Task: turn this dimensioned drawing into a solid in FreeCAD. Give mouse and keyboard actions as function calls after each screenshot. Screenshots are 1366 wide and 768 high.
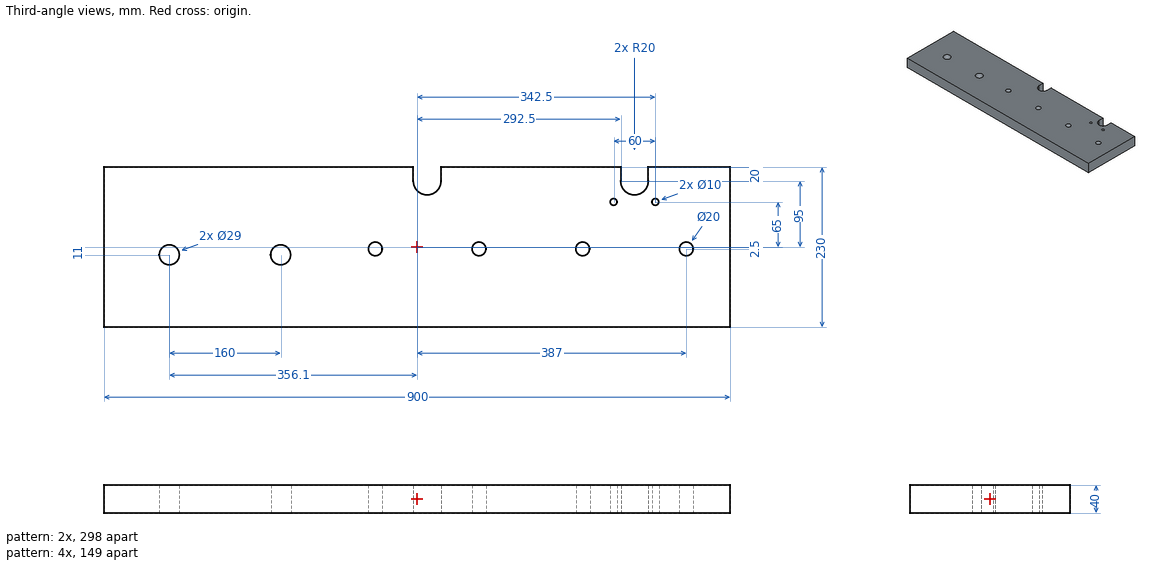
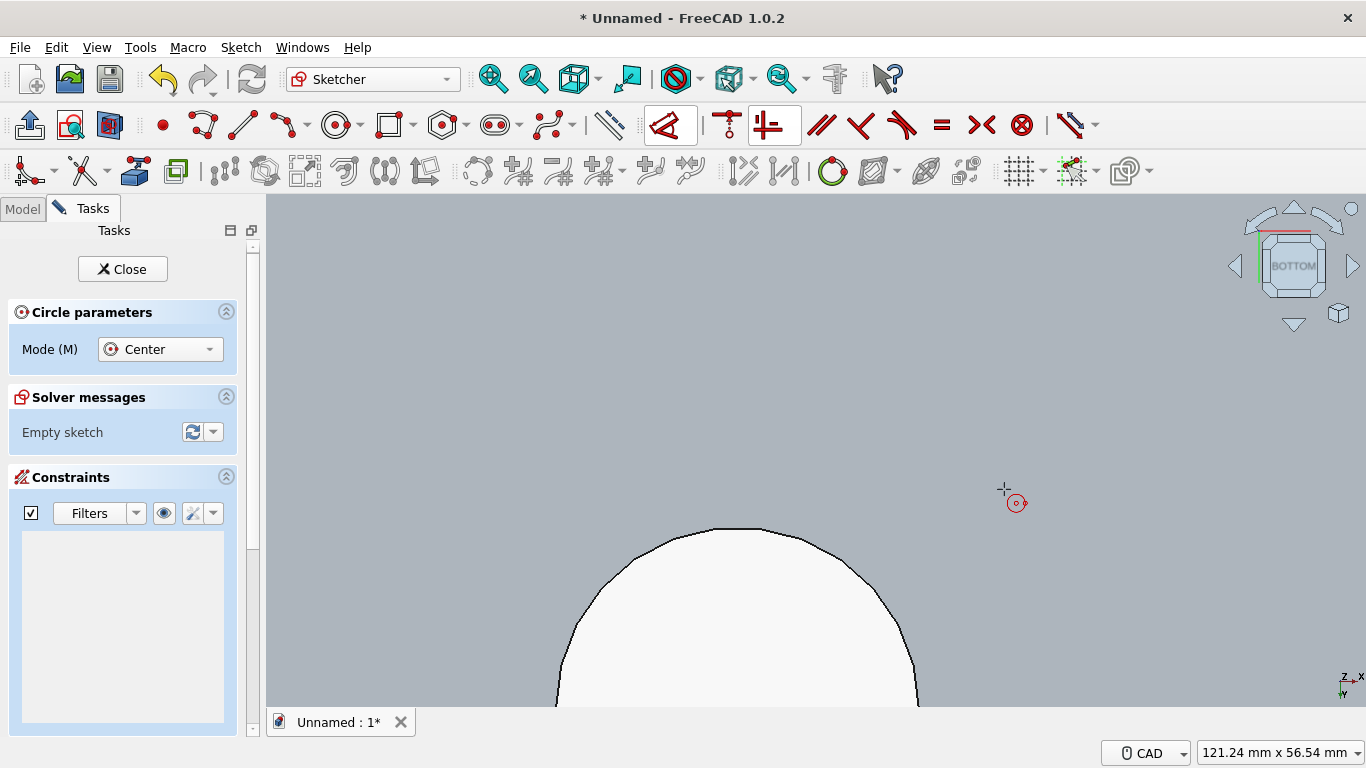
click(1010, 437)
move(1042, 405)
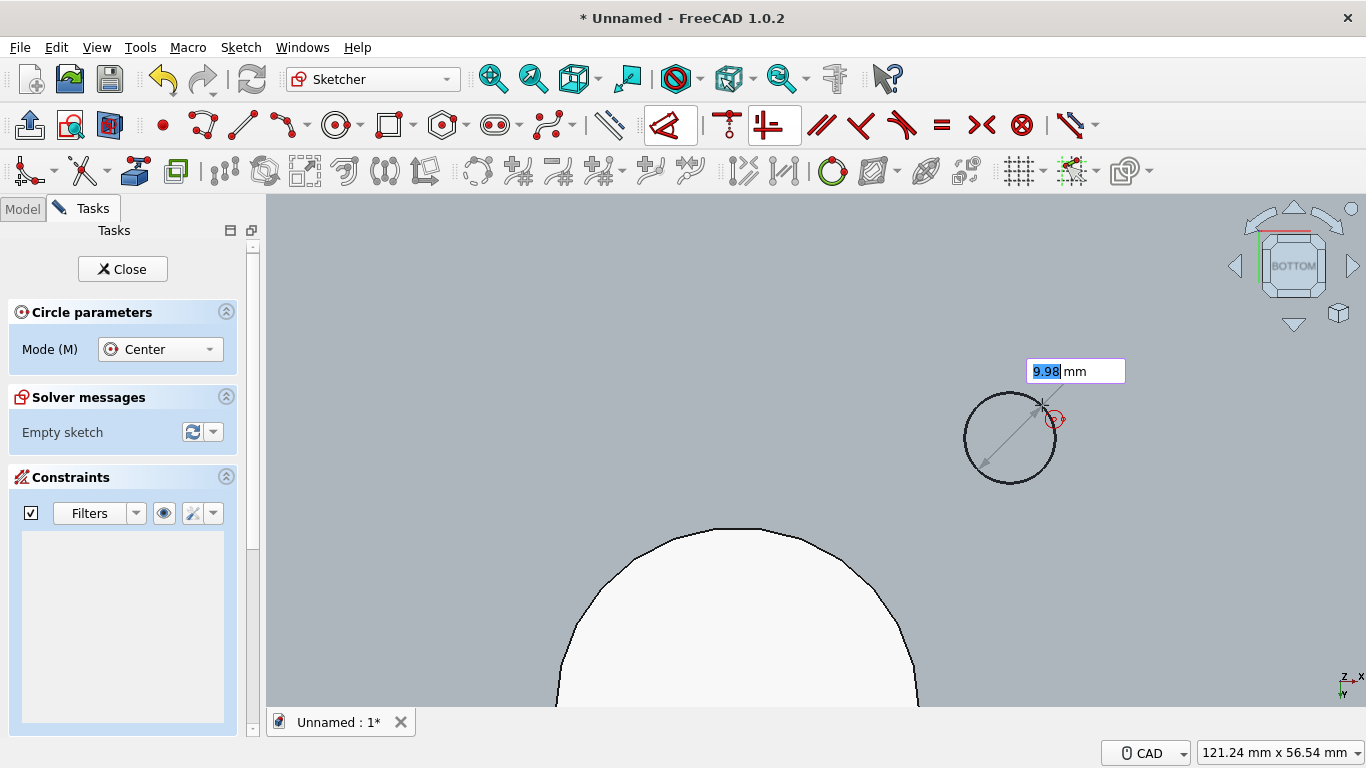
text(10)
key(Return)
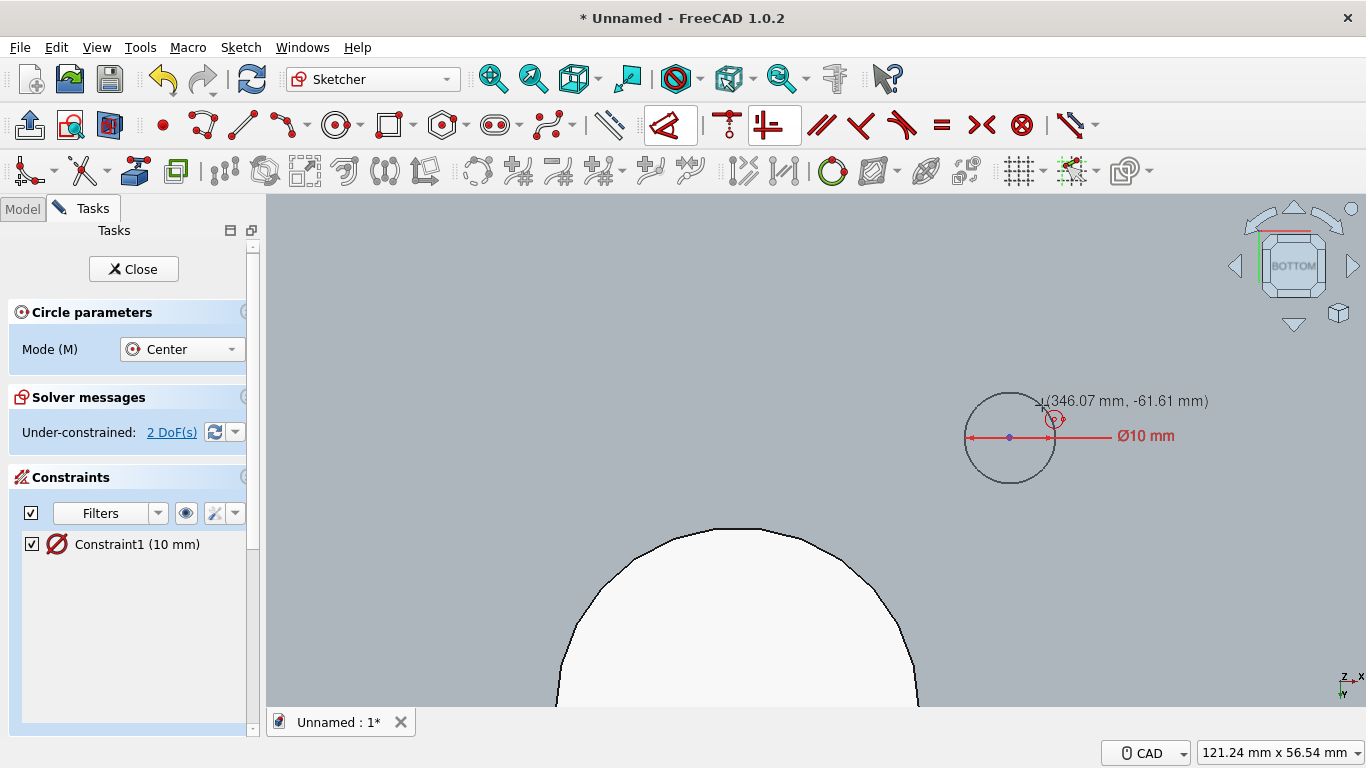
click(465, 437)
move(497, 405)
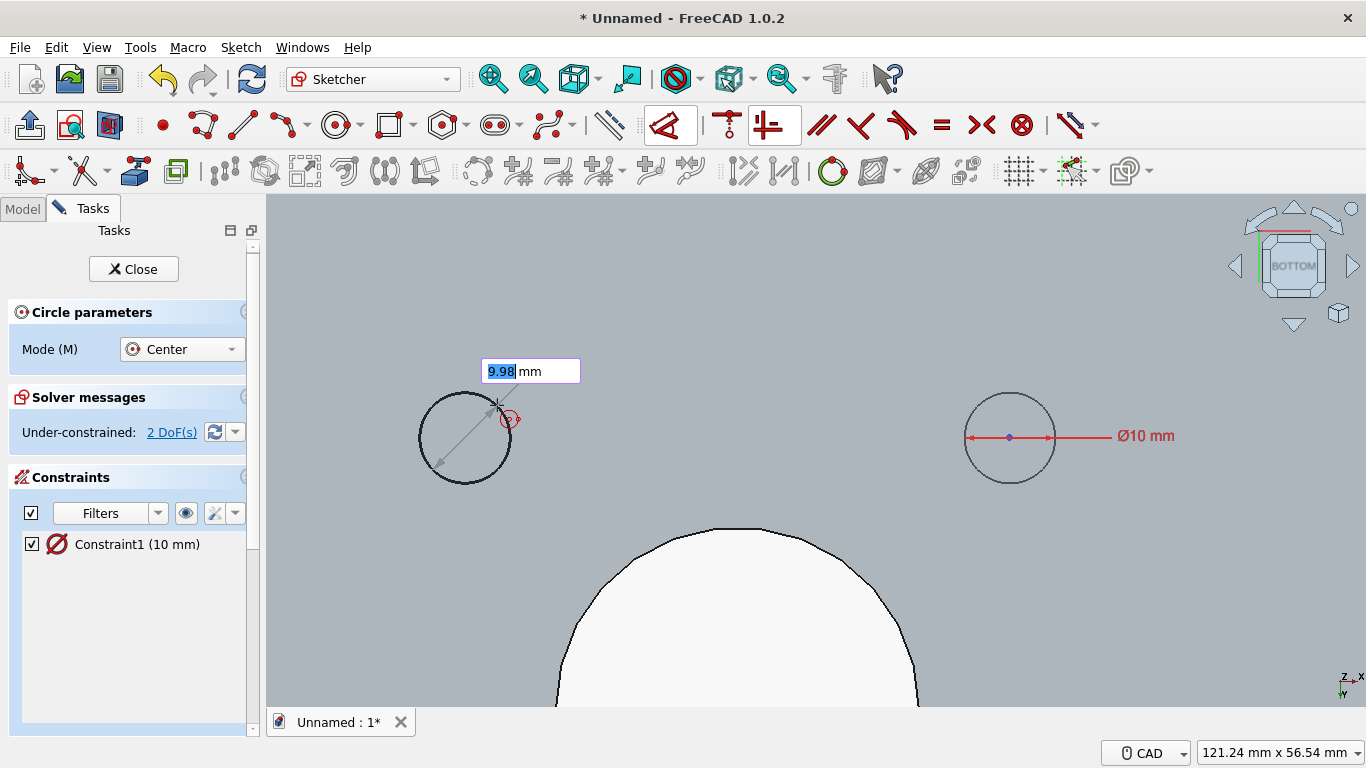
text(10)
key(Return)
key(Escape)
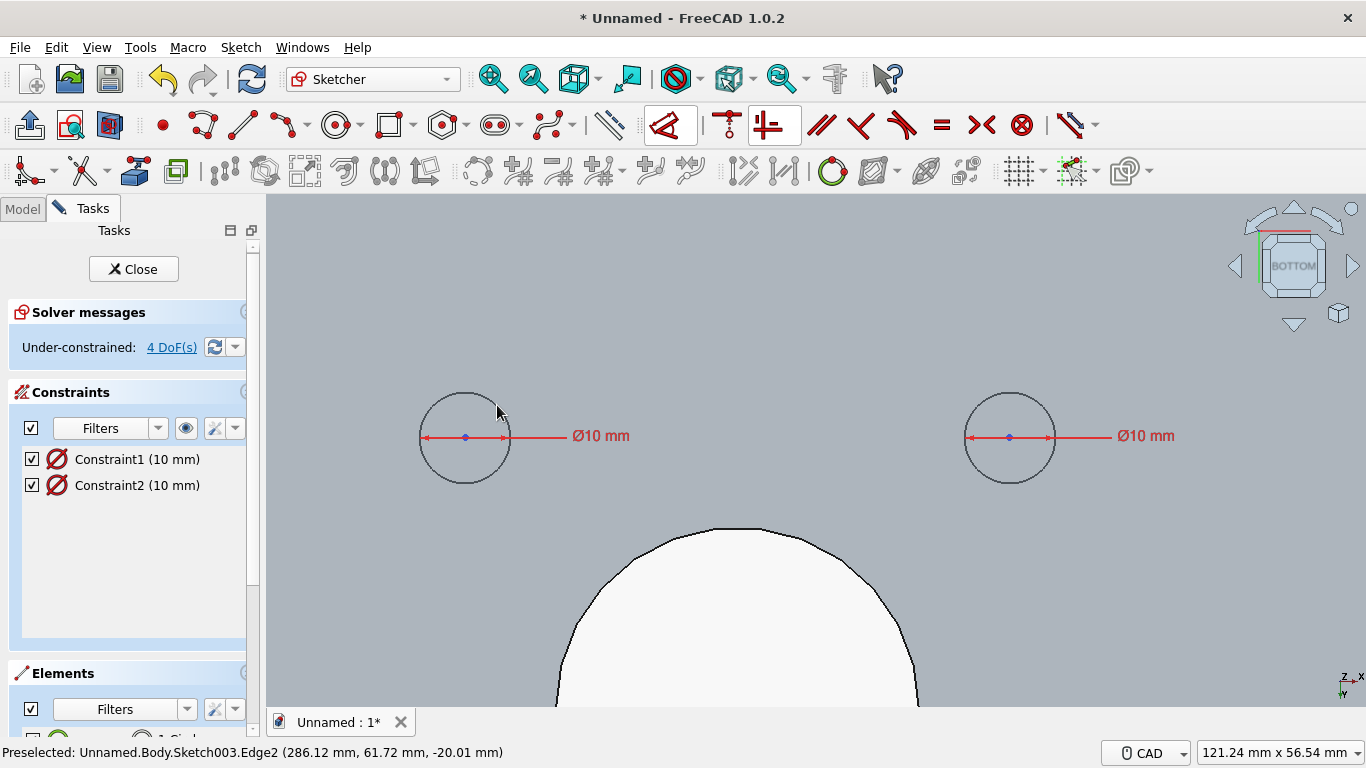
click(1010, 438)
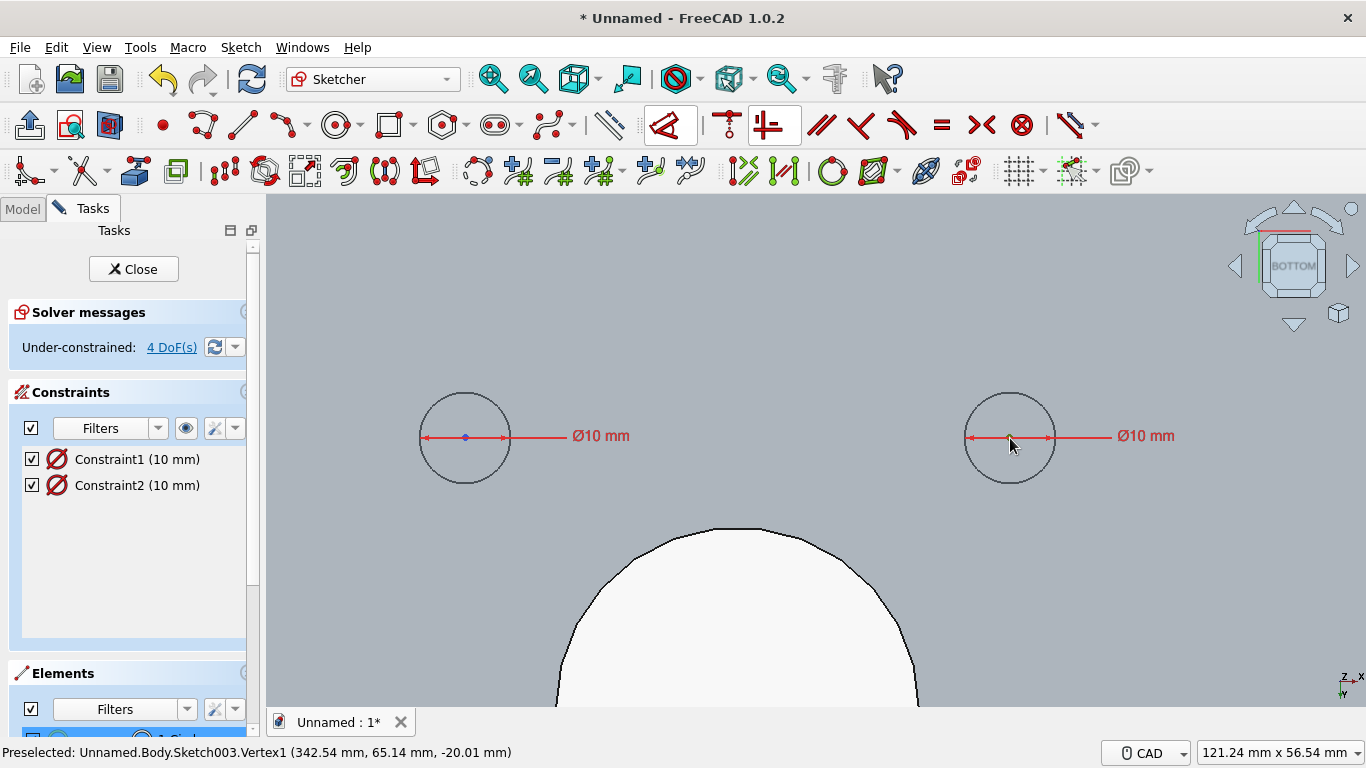
click(465, 438)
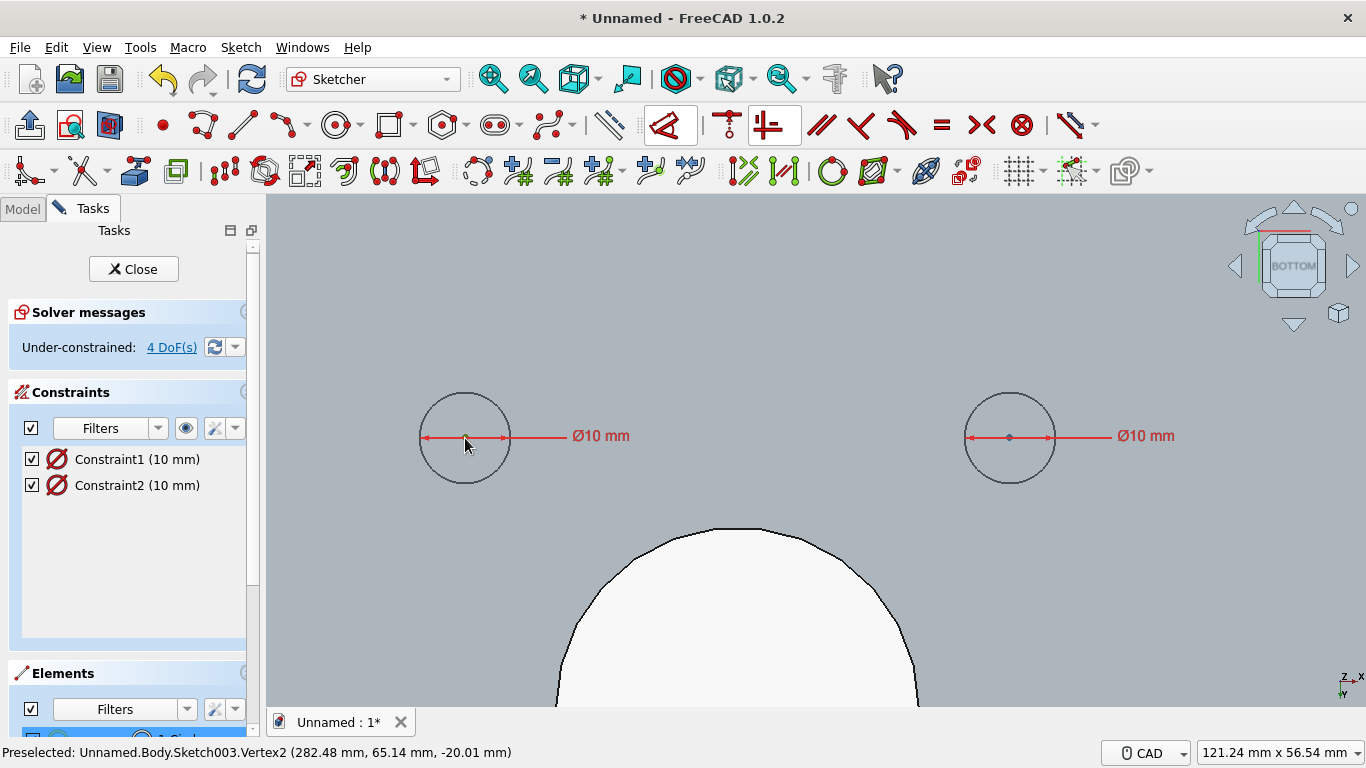
click(796, 126)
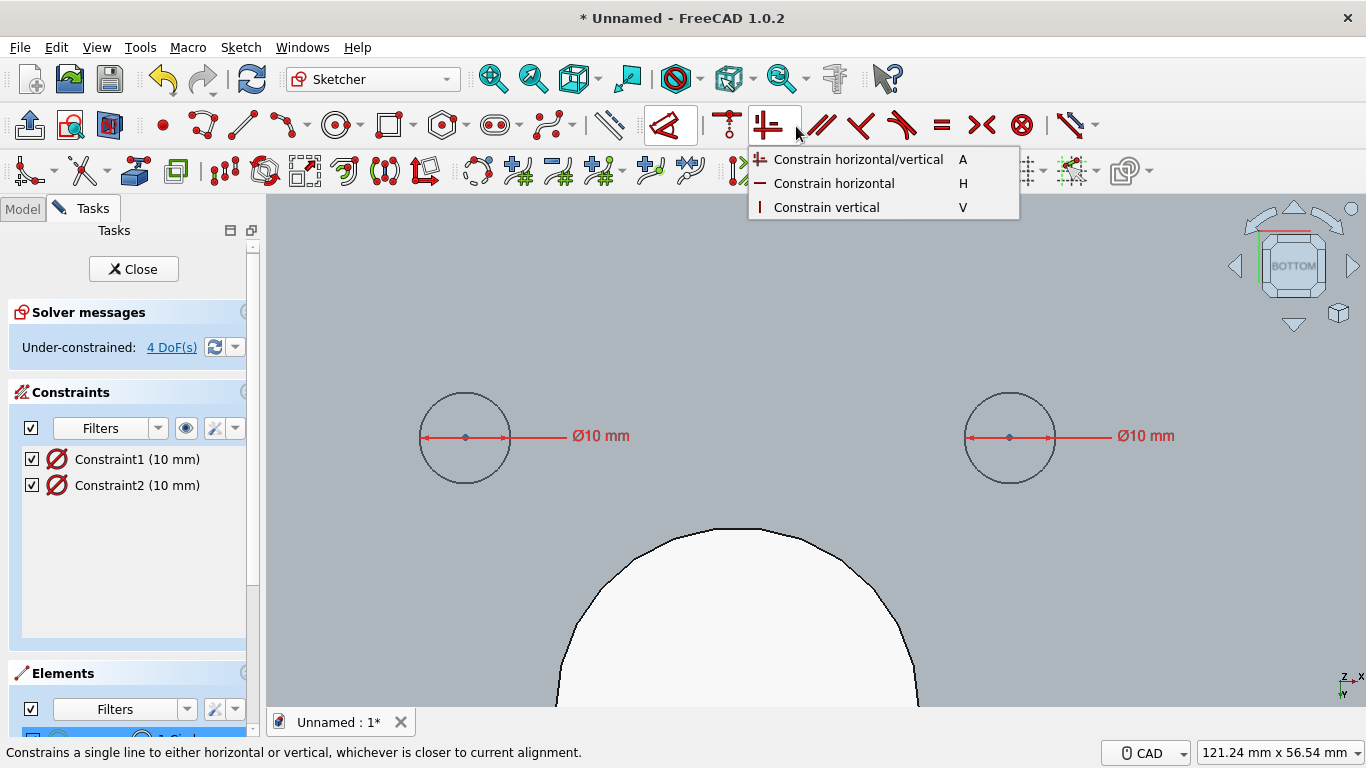
click(884, 183)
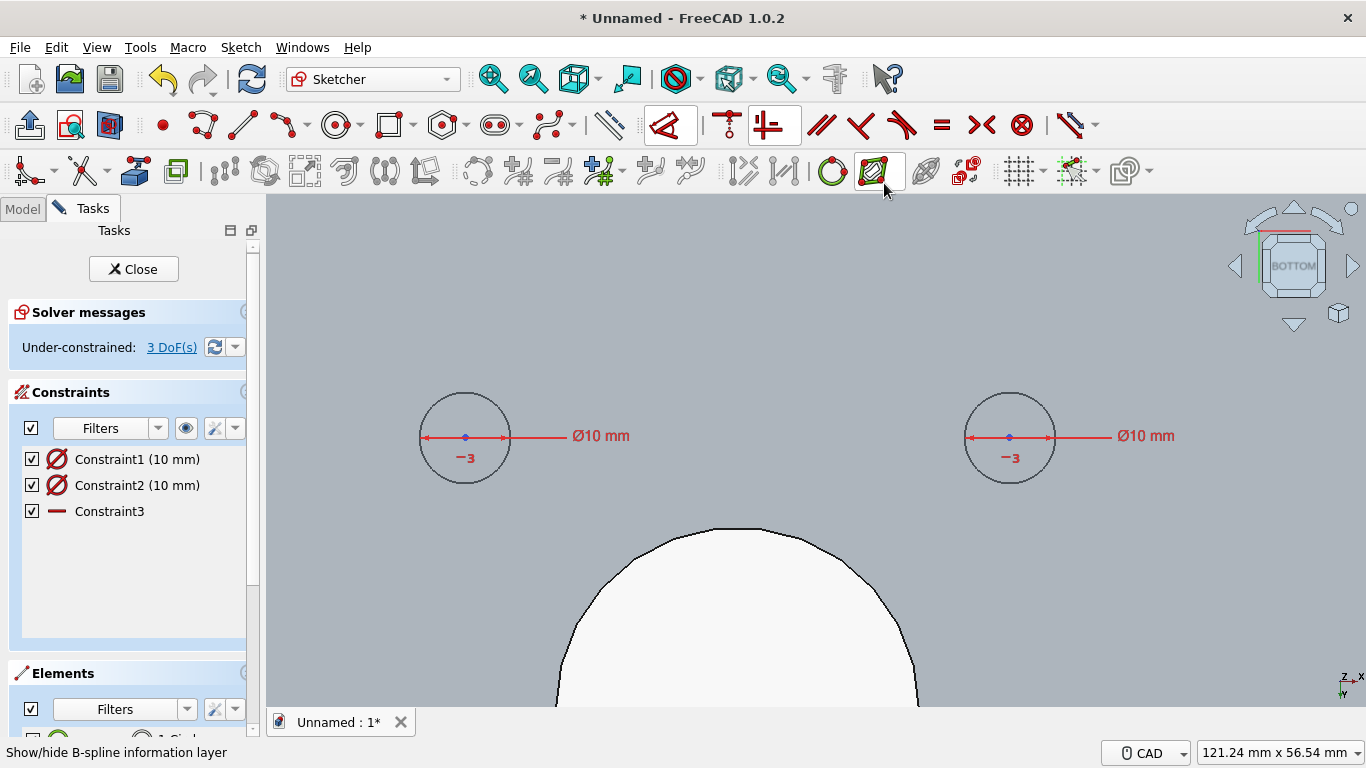
click(1010, 438)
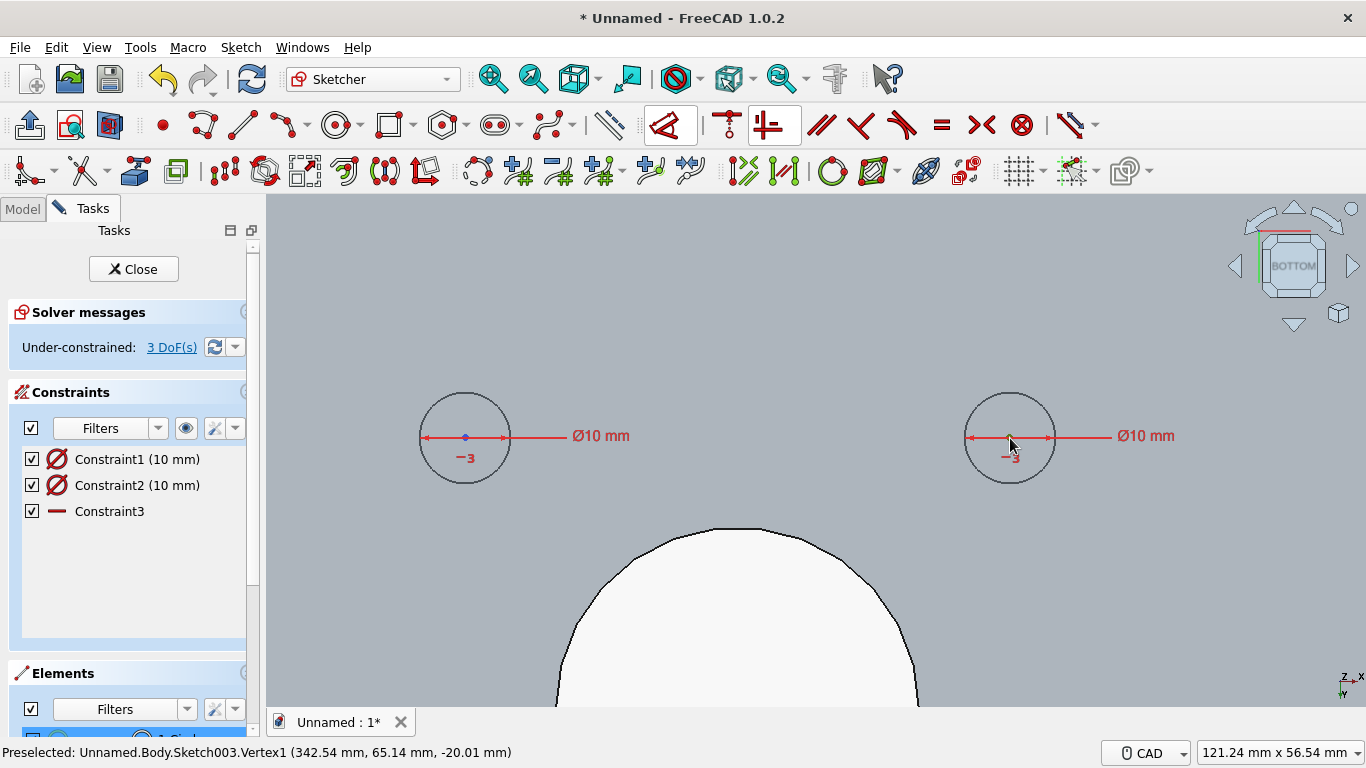
key(i)